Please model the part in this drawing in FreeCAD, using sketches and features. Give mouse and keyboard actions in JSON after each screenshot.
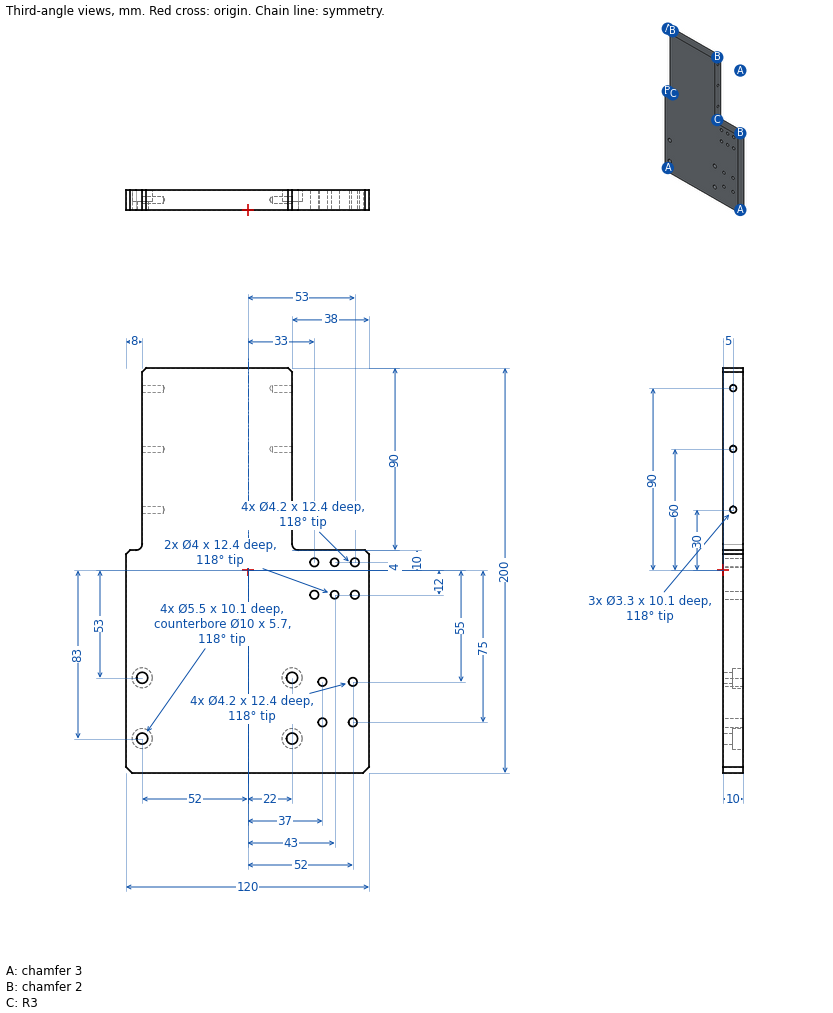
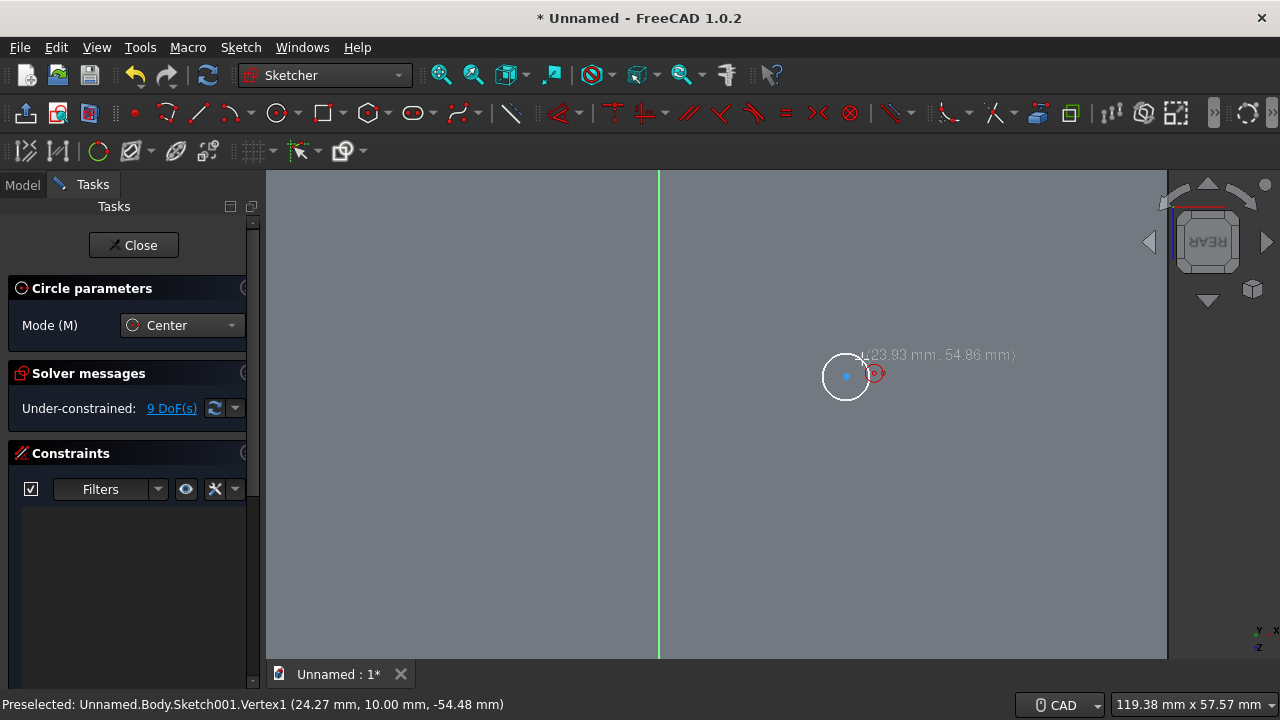
{"action": "scroll", "coordinate": [846, 376], "scroll_direction": "down", "scroll_amount": 4}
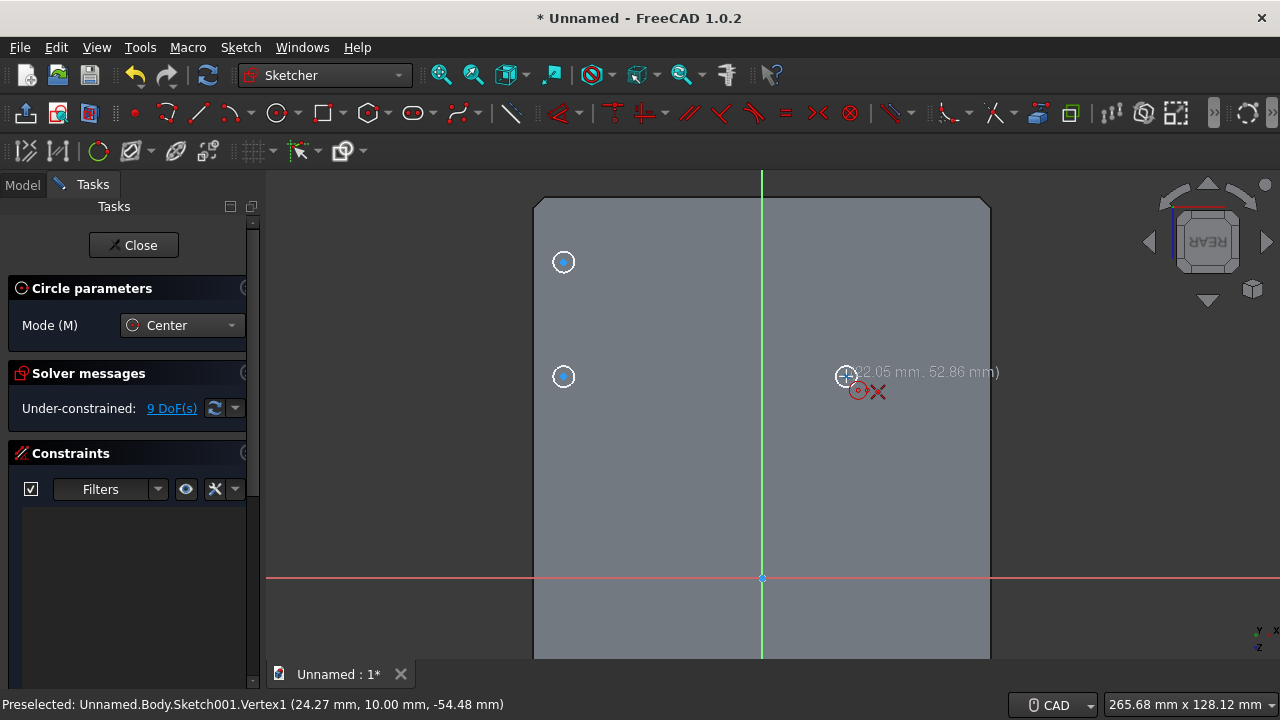
{"action": "scroll", "coordinate": [846, 262], "scroll_direction": "up", "scroll_amount": 4}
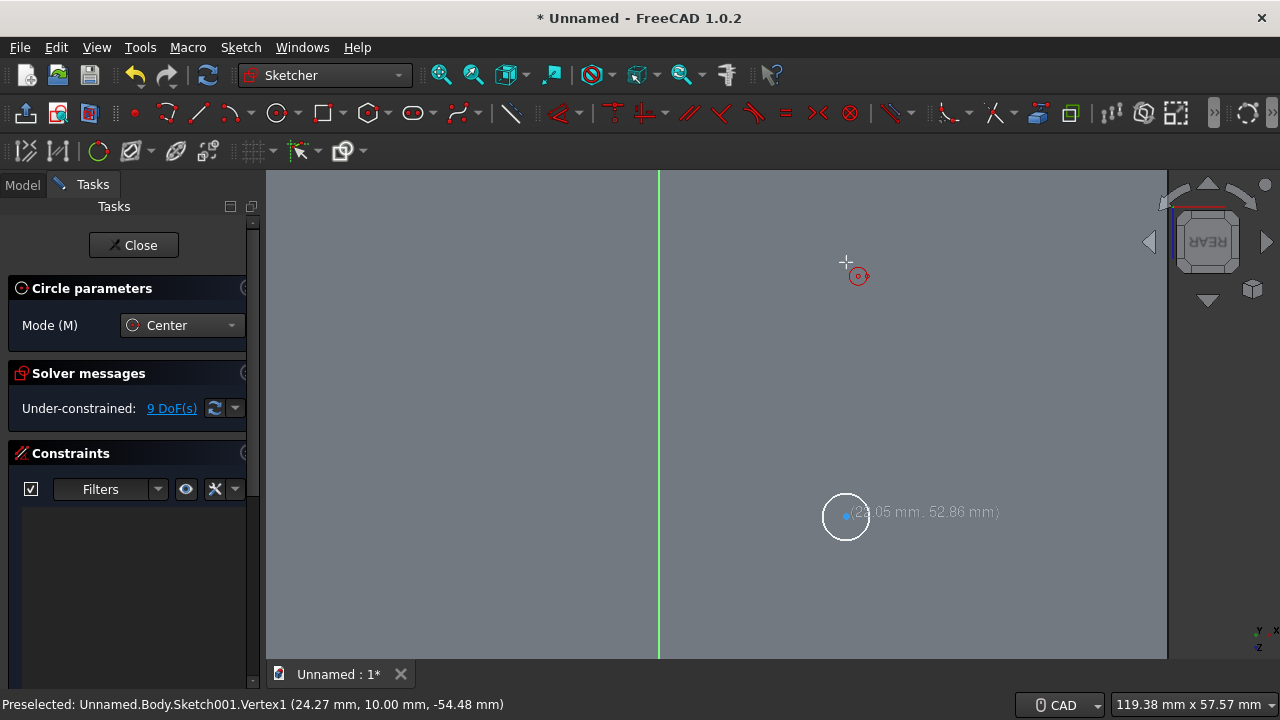
{"action": "left_click", "coordinate": [846, 261]}
{"action": "left_click", "coordinate": [862, 244]}
{"action": "key", "text": "Escape"}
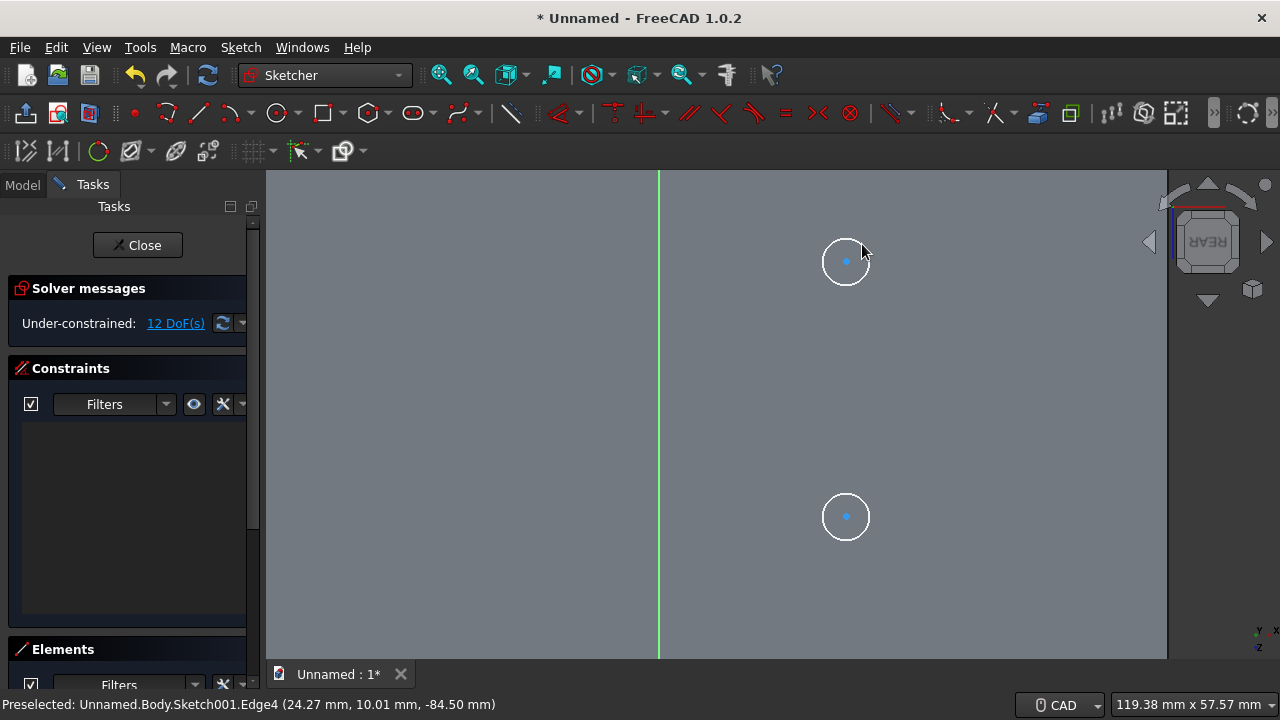
{"action": "scroll", "coordinate": [846, 262], "scroll_direction": "down", "scroll_amount": 4}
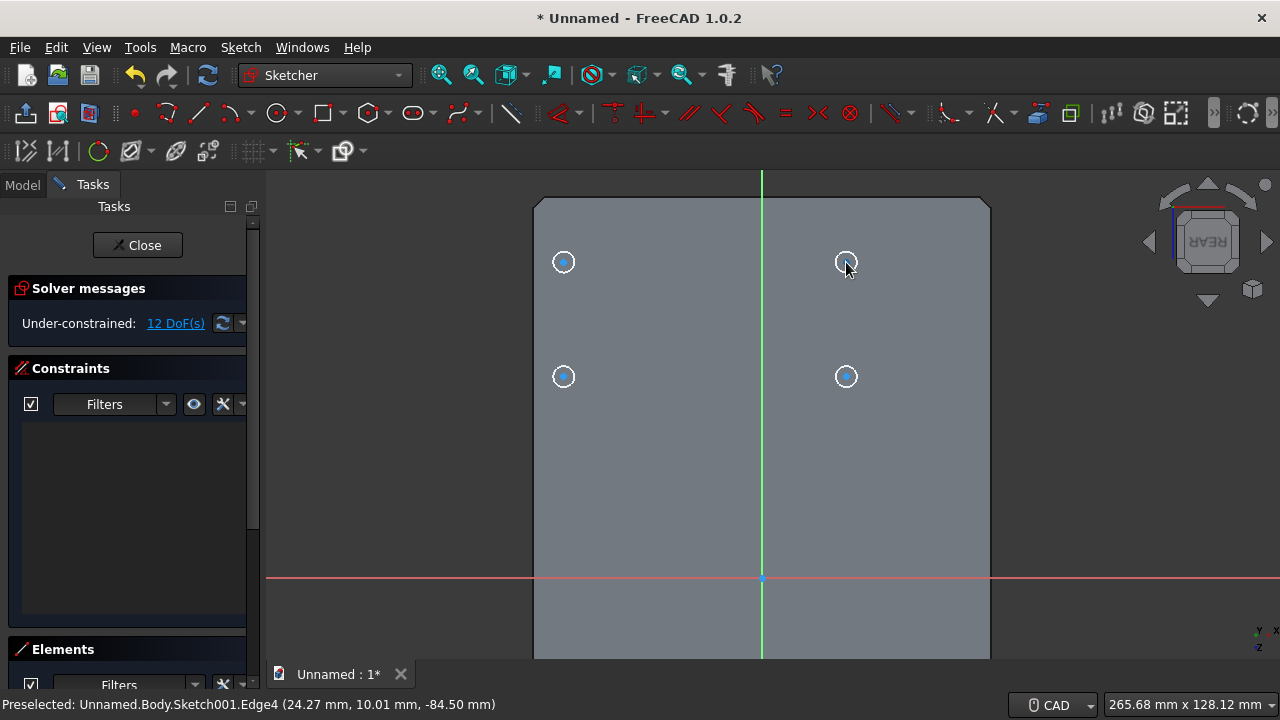
{"action": "scroll", "coordinate": [571, 255], "scroll_direction": "up", "scroll_amount": 2}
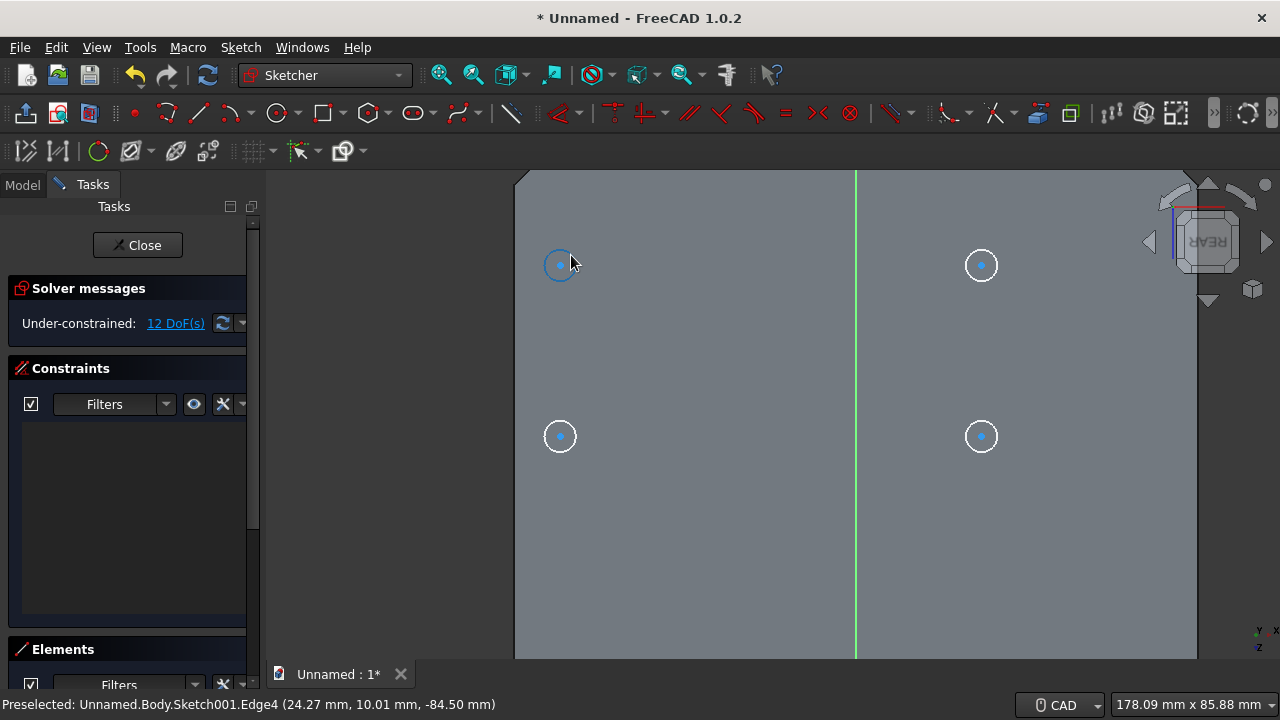
{"action": "left_click", "coordinate": [571, 254]}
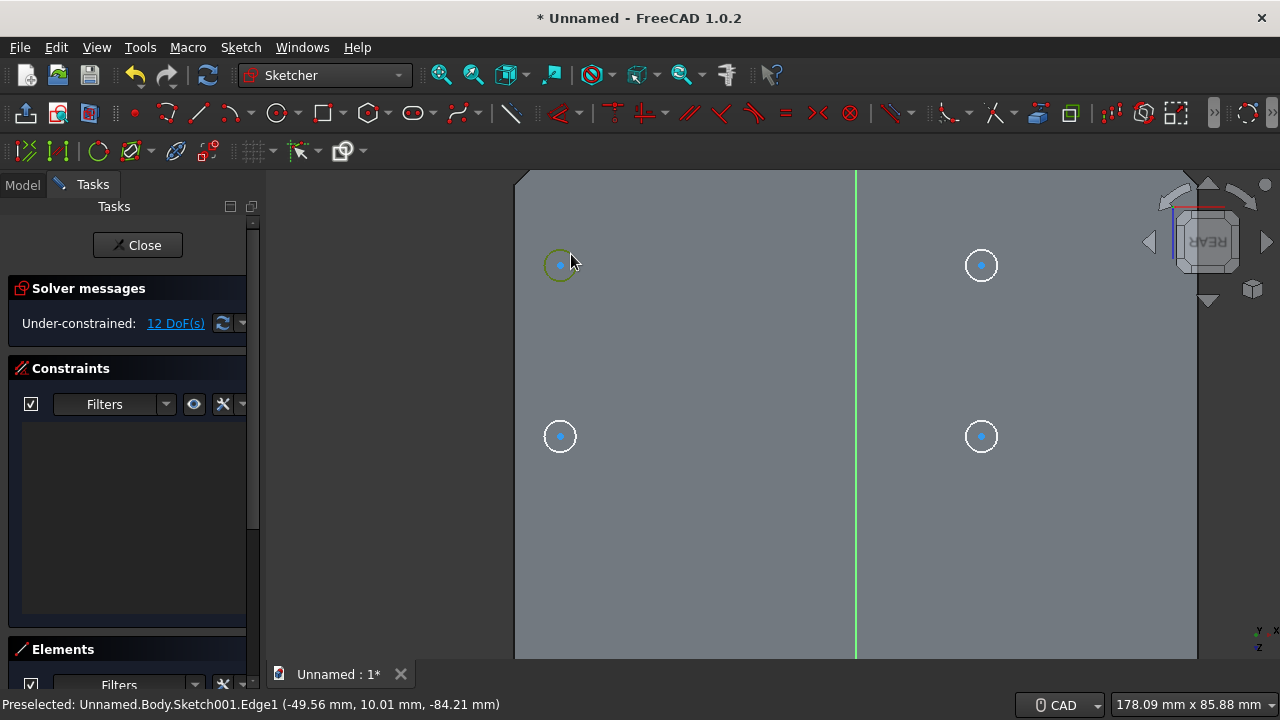
{"action": "left_click", "coordinate": [571, 425]}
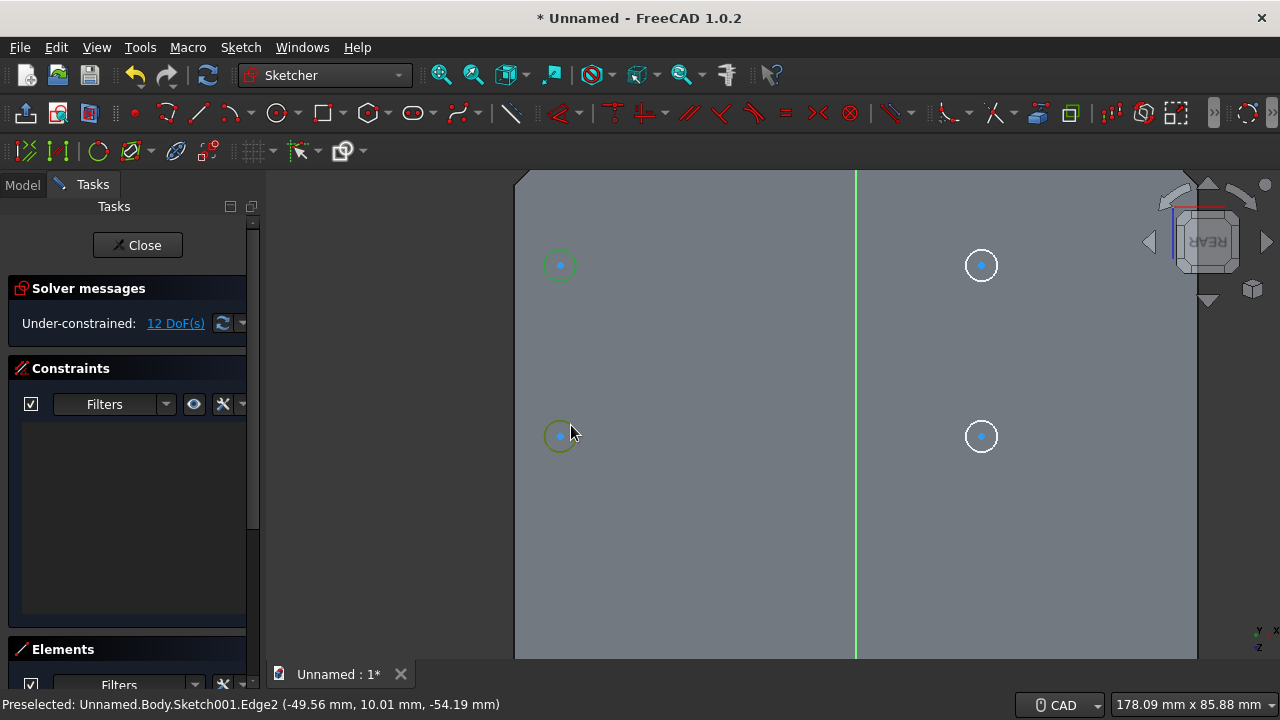
{"action": "left_click", "coordinate": [993, 425]}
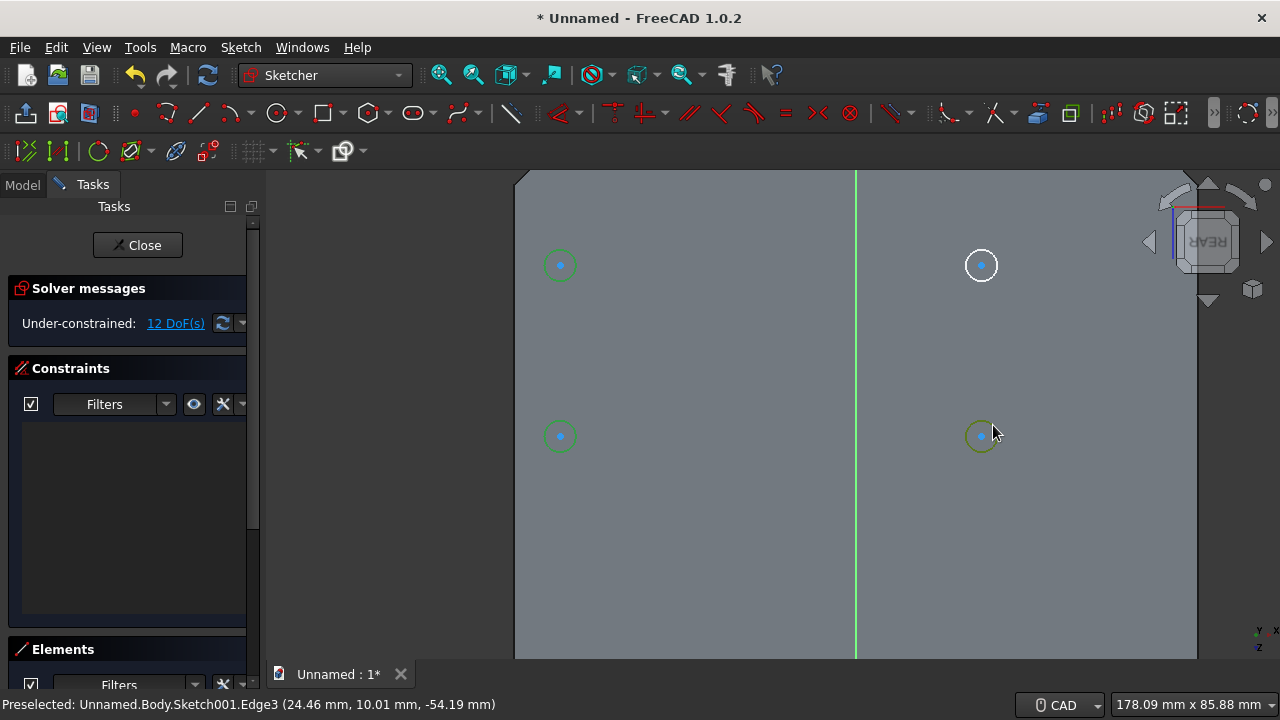
{"action": "left_click", "coordinate": [993, 254]}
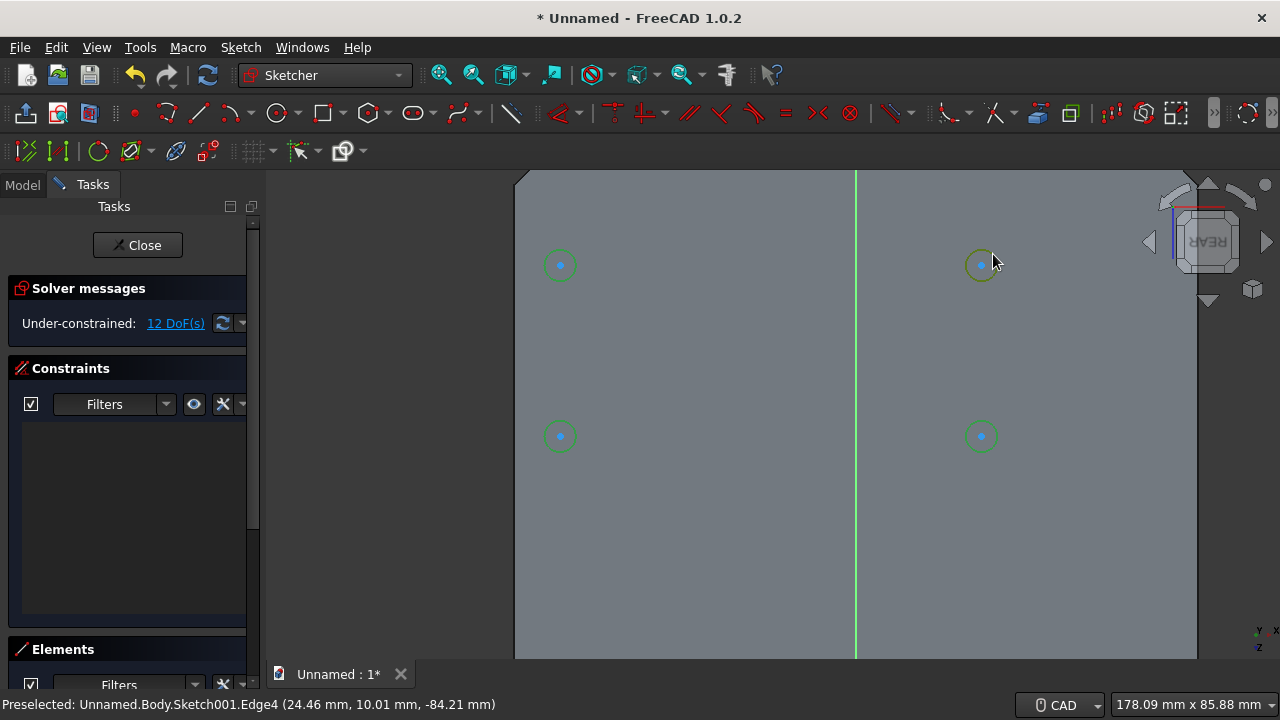
{"action": "key", "text": "e"}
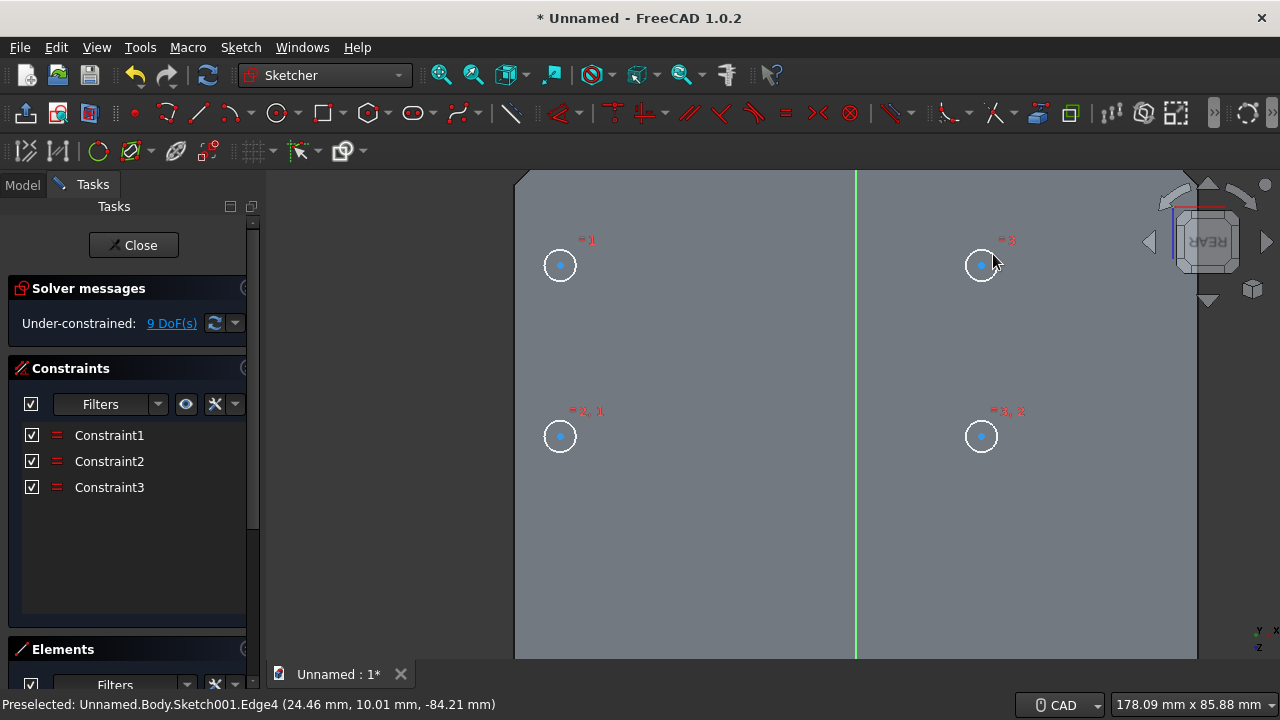
{"action": "left_click", "coordinate": [560, 266]}